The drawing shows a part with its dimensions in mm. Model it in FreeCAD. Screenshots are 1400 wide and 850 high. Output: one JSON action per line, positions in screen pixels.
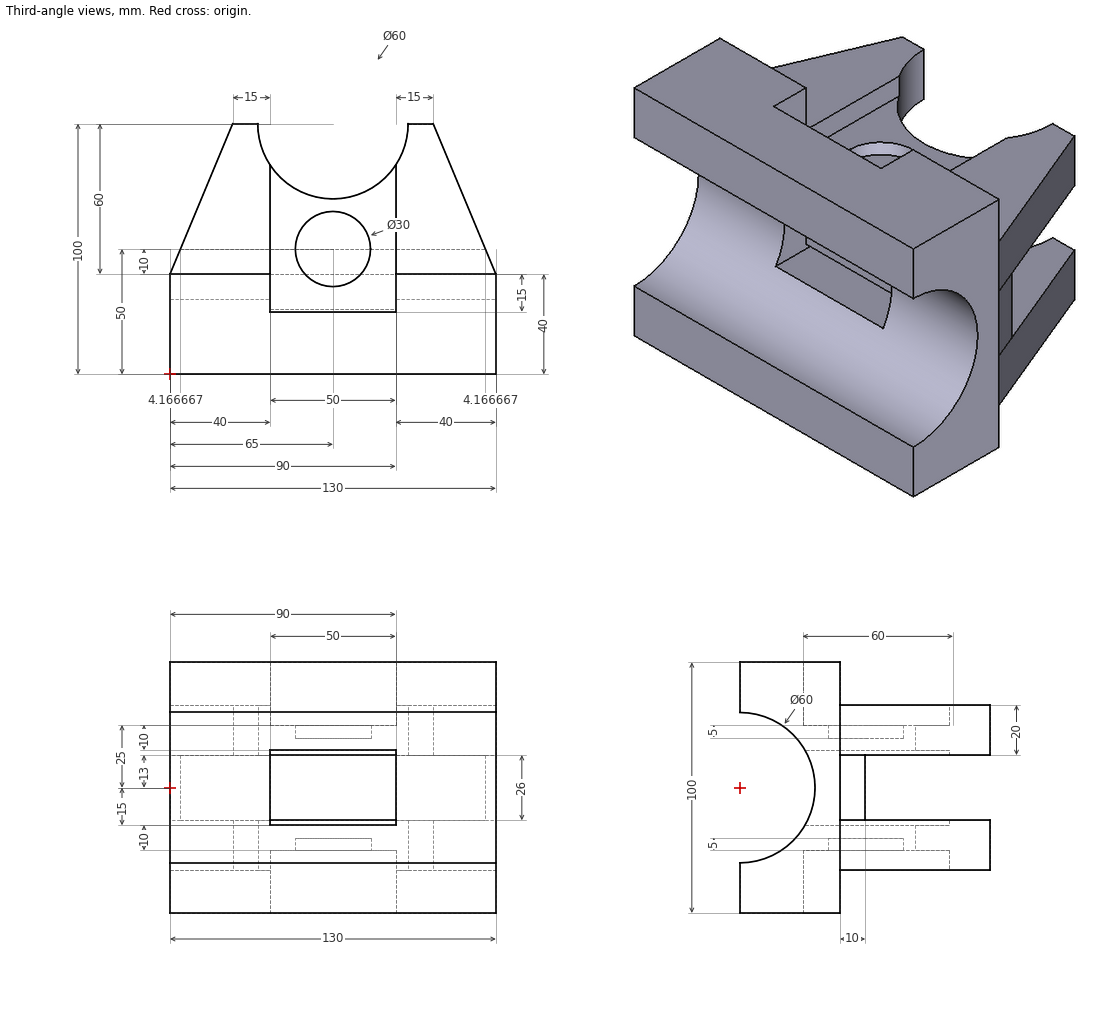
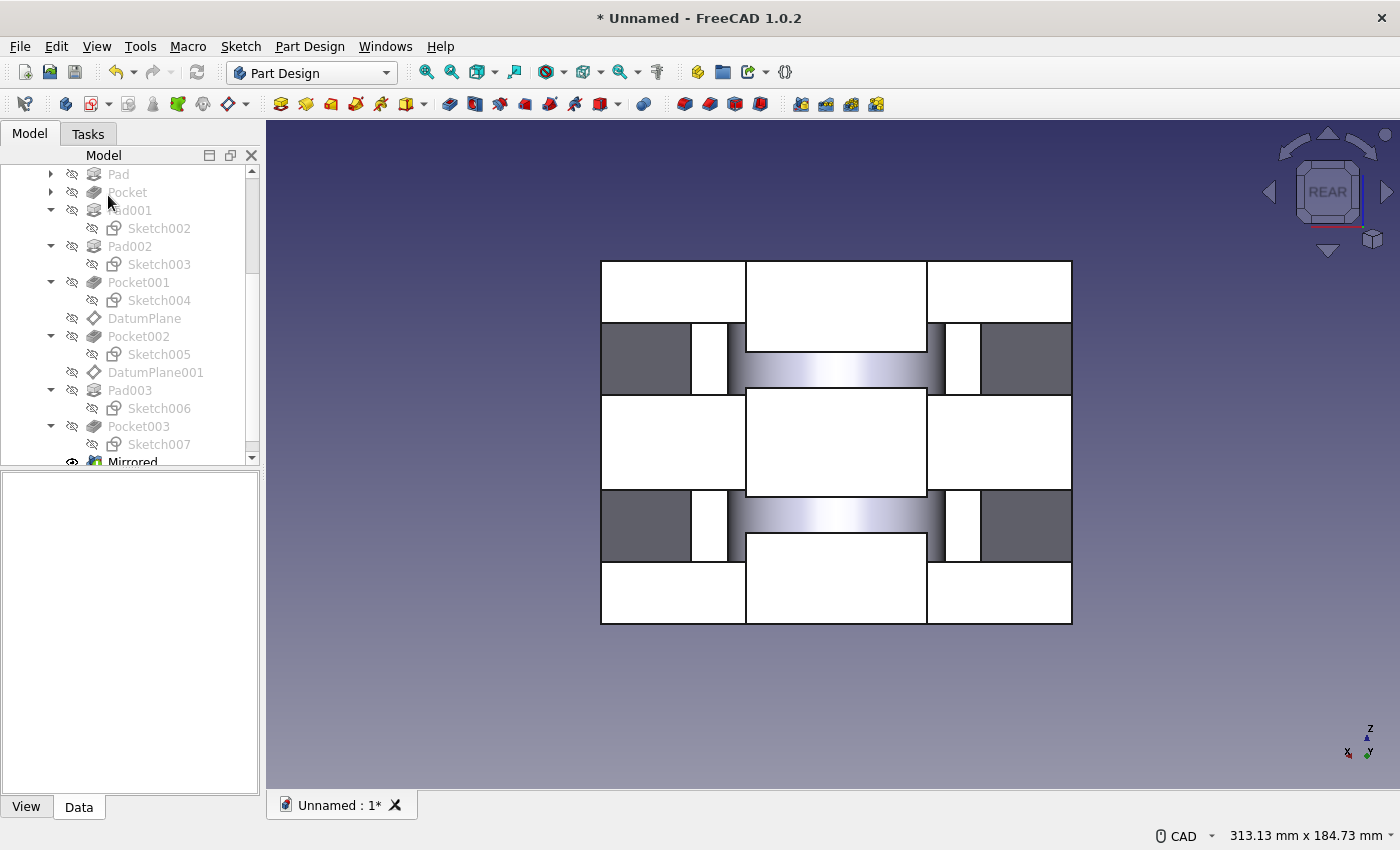
{"action": "left_click", "coordinate": [979, 442]}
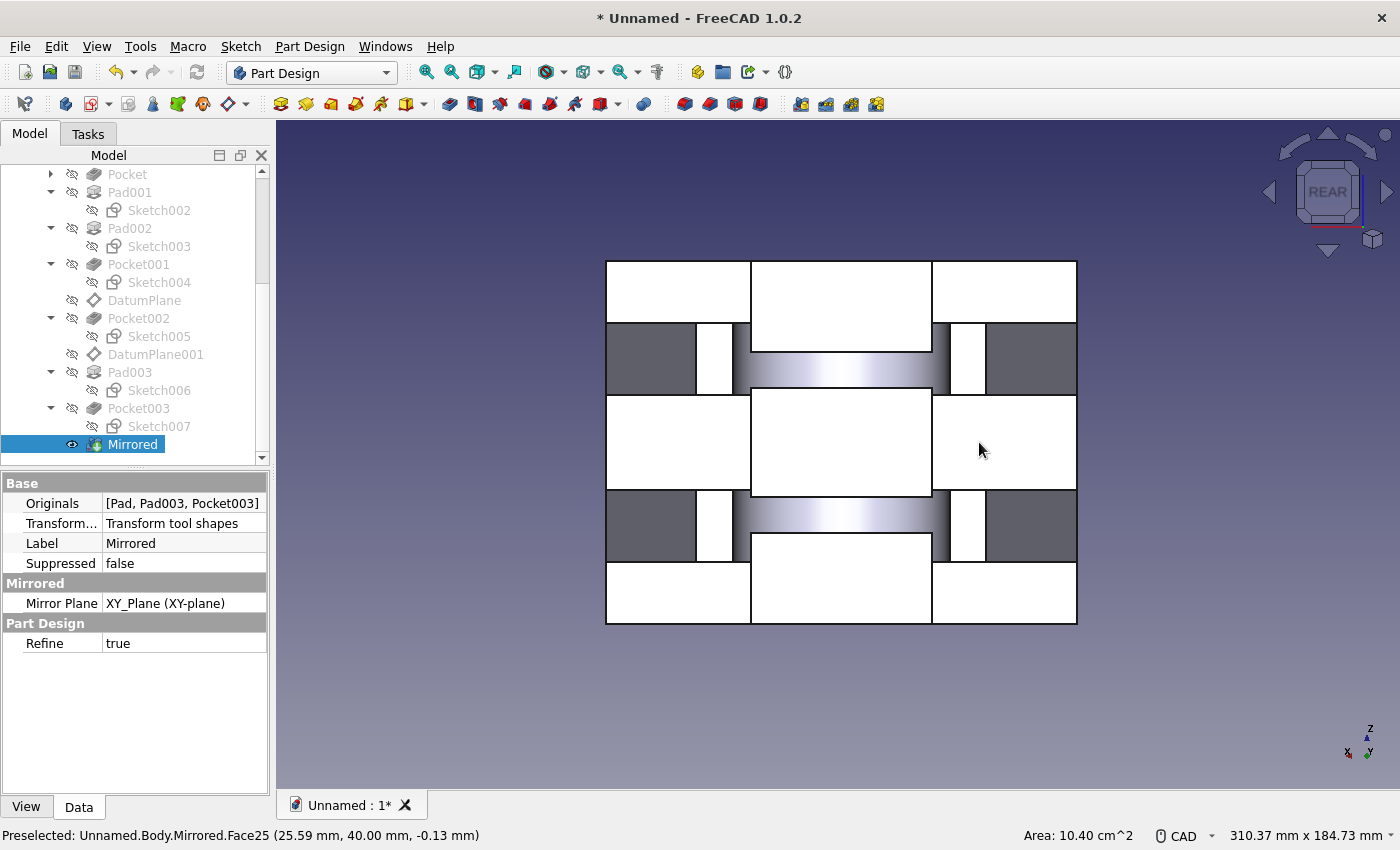
{"action": "left_click", "coordinate": [90, 104]}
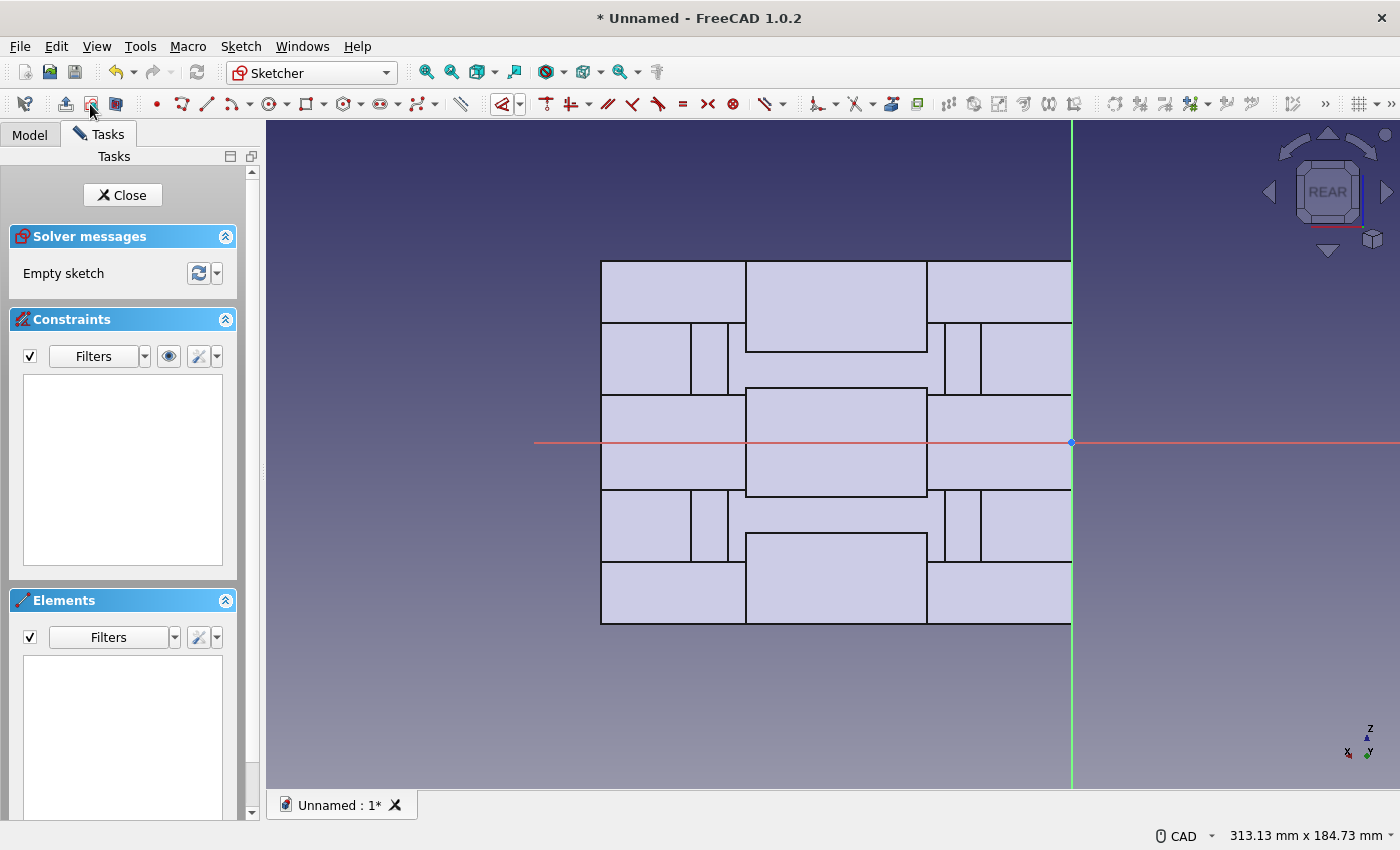
{"action": "left_click", "coordinate": [116, 104]}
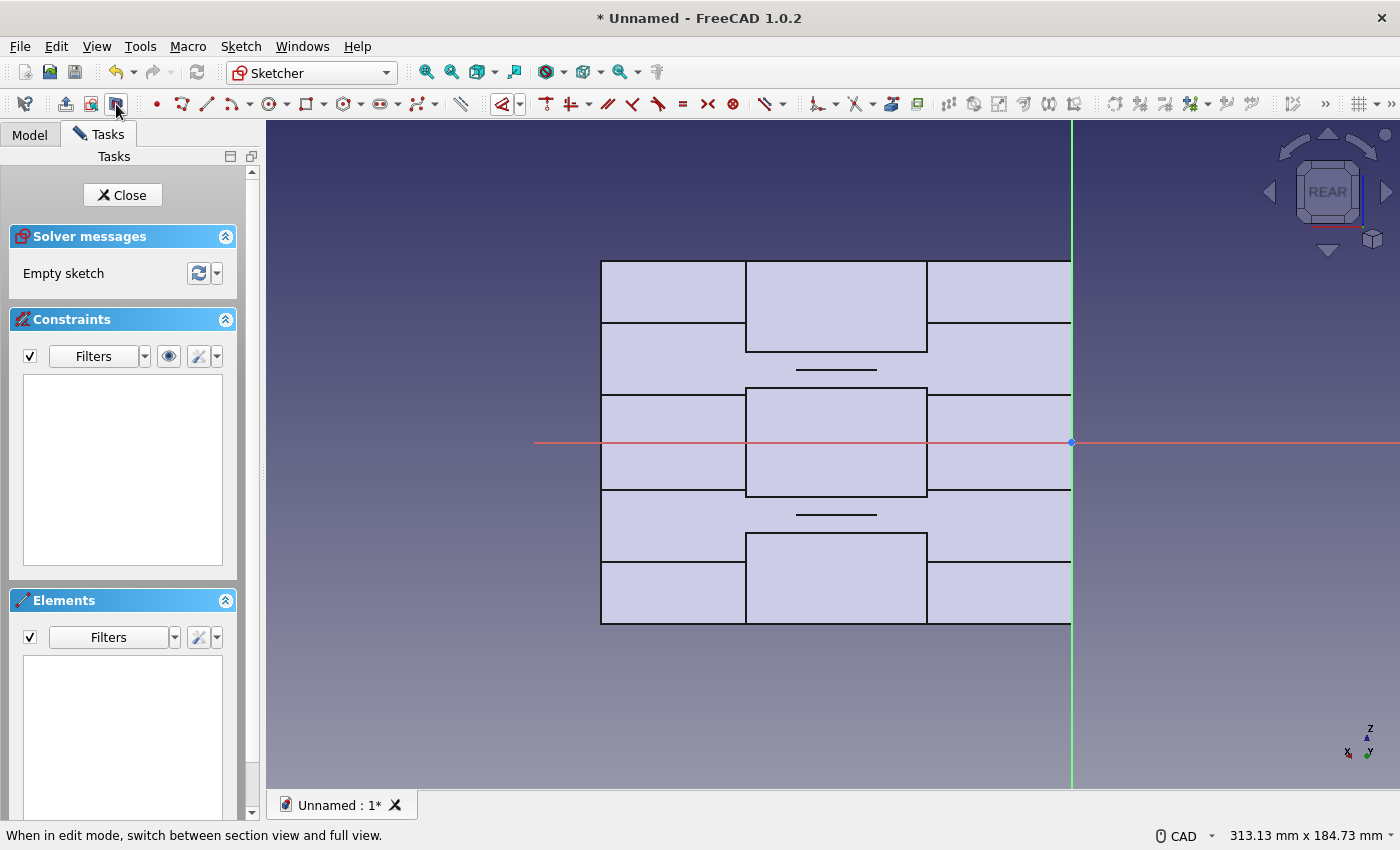
{"action": "scroll", "coordinate": [982, 418], "scroll_direction": "up", "scroll_amount": 2}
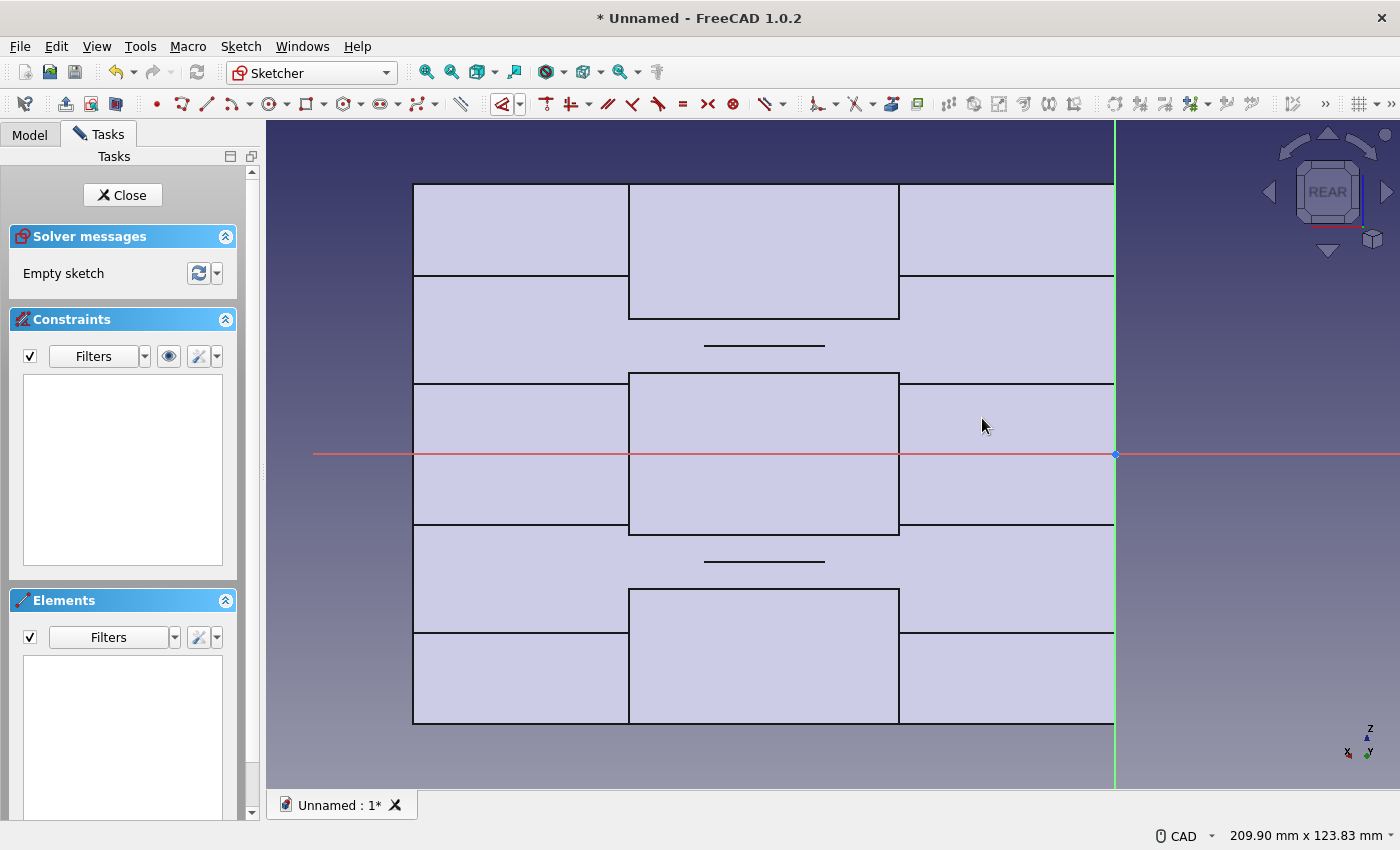
{"action": "left_click", "coordinate": [306, 104]}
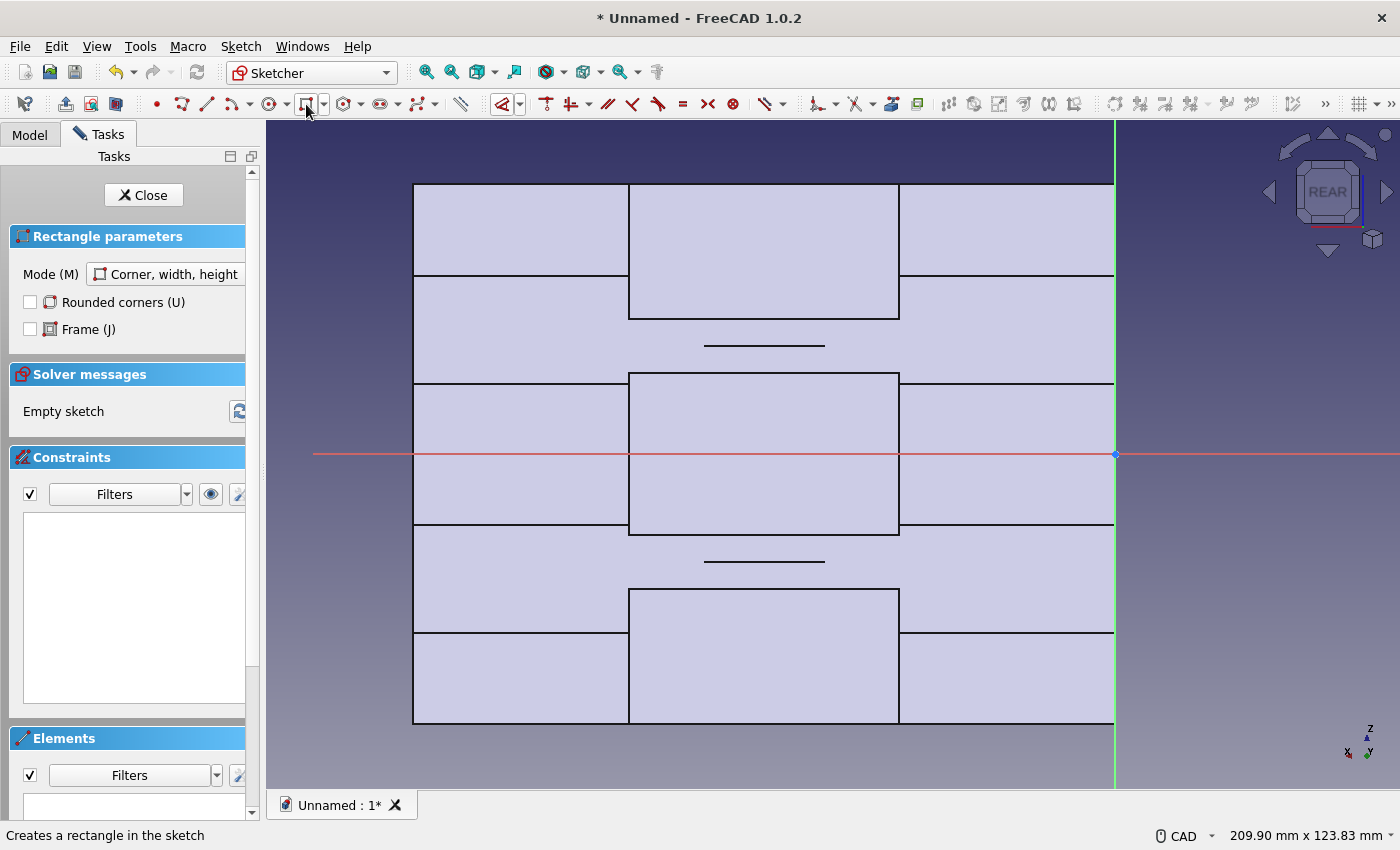
{"action": "left_click", "coordinate": [413, 384]}
{"action": "left_click", "coordinate": [1115, 525]}
{"action": "key", "text": "Escape"}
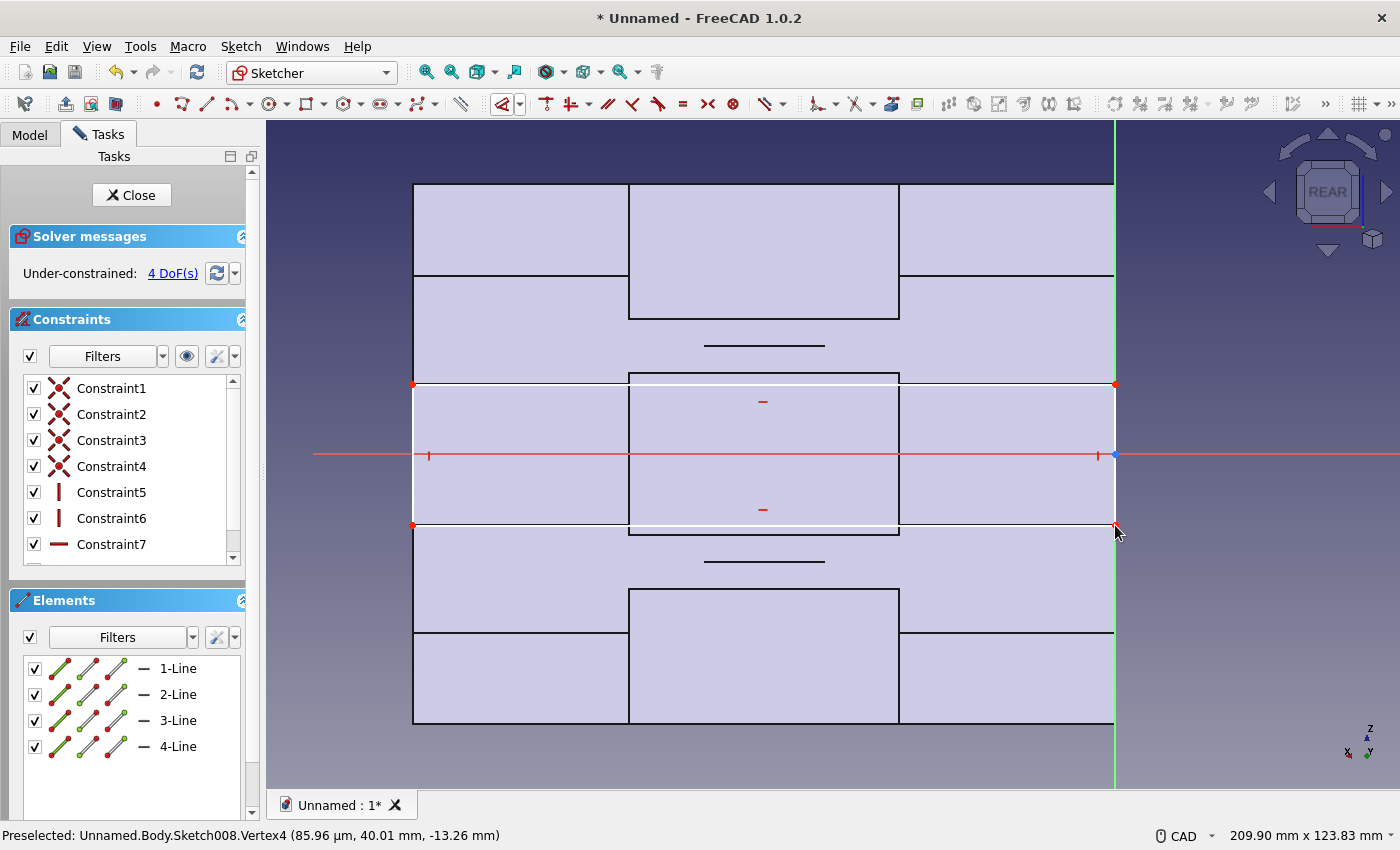
{"action": "left_click", "coordinate": [1115, 526]}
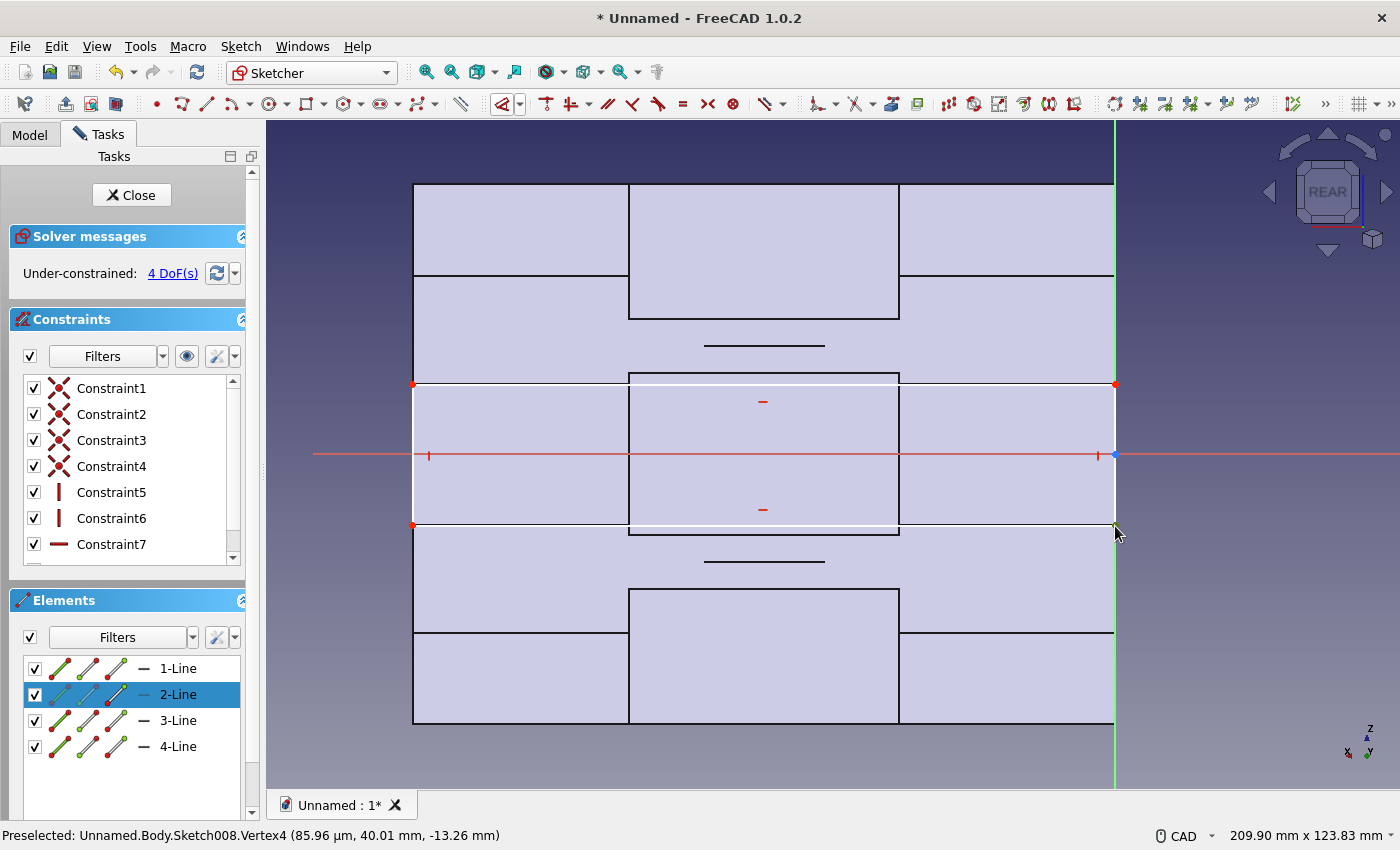
{"action": "left_click", "coordinate": [1115, 717]}